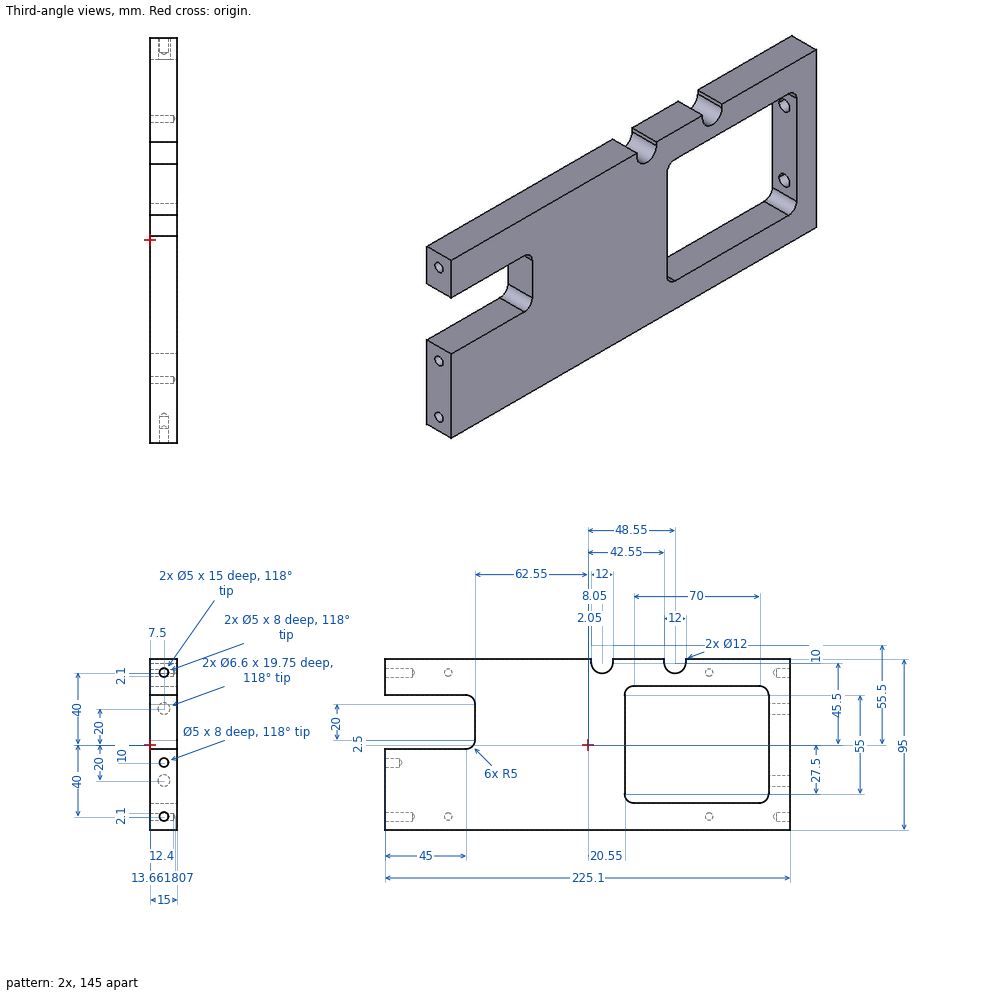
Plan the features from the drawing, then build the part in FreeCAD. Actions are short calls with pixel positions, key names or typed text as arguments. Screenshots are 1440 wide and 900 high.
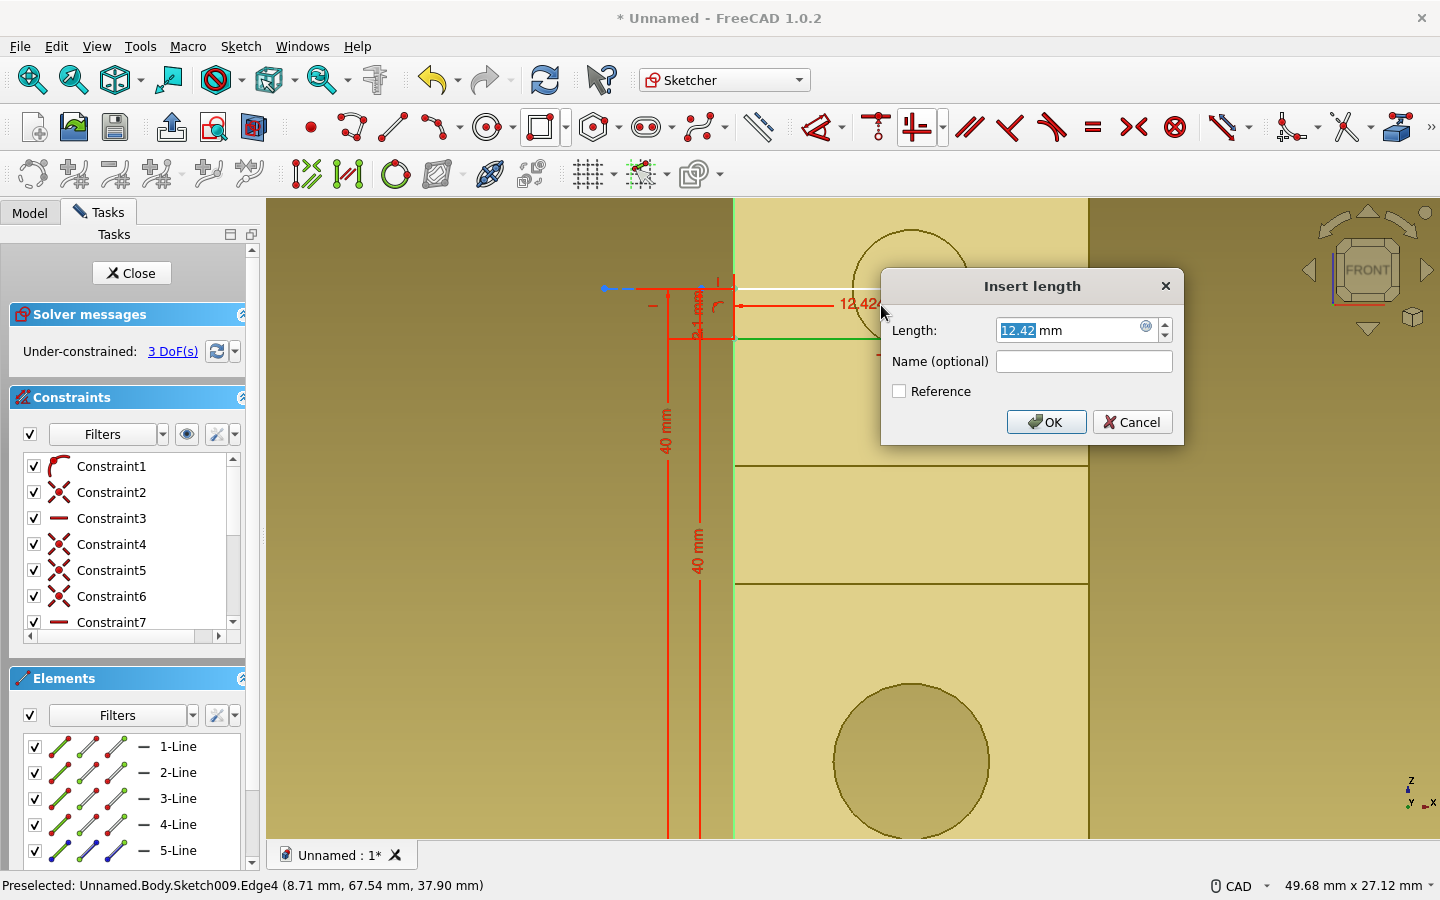
text(12.4)
key(Return)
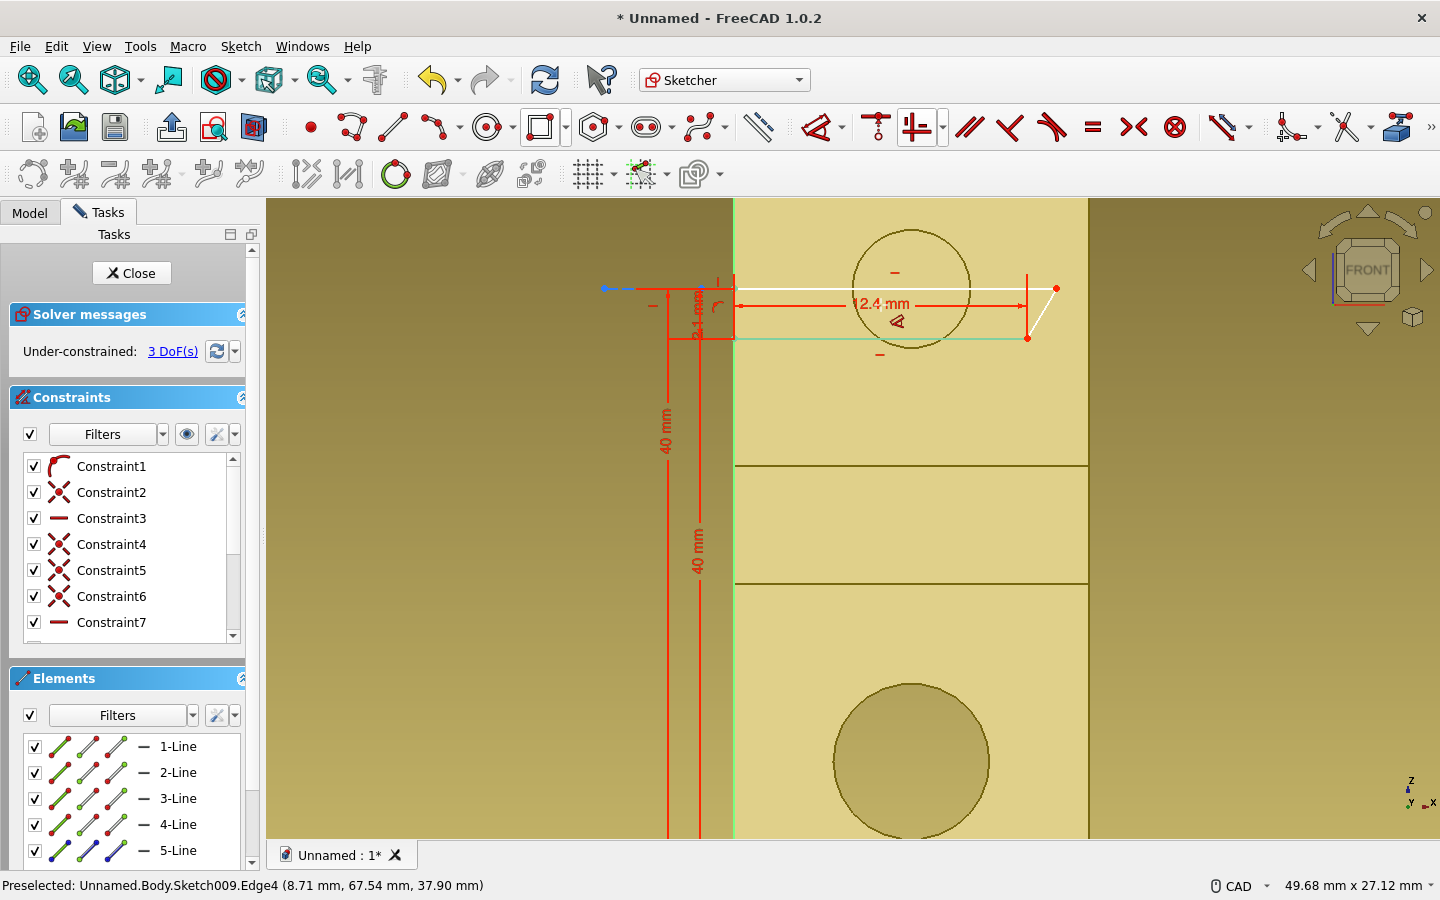
click(831, 289)
click(895, 255)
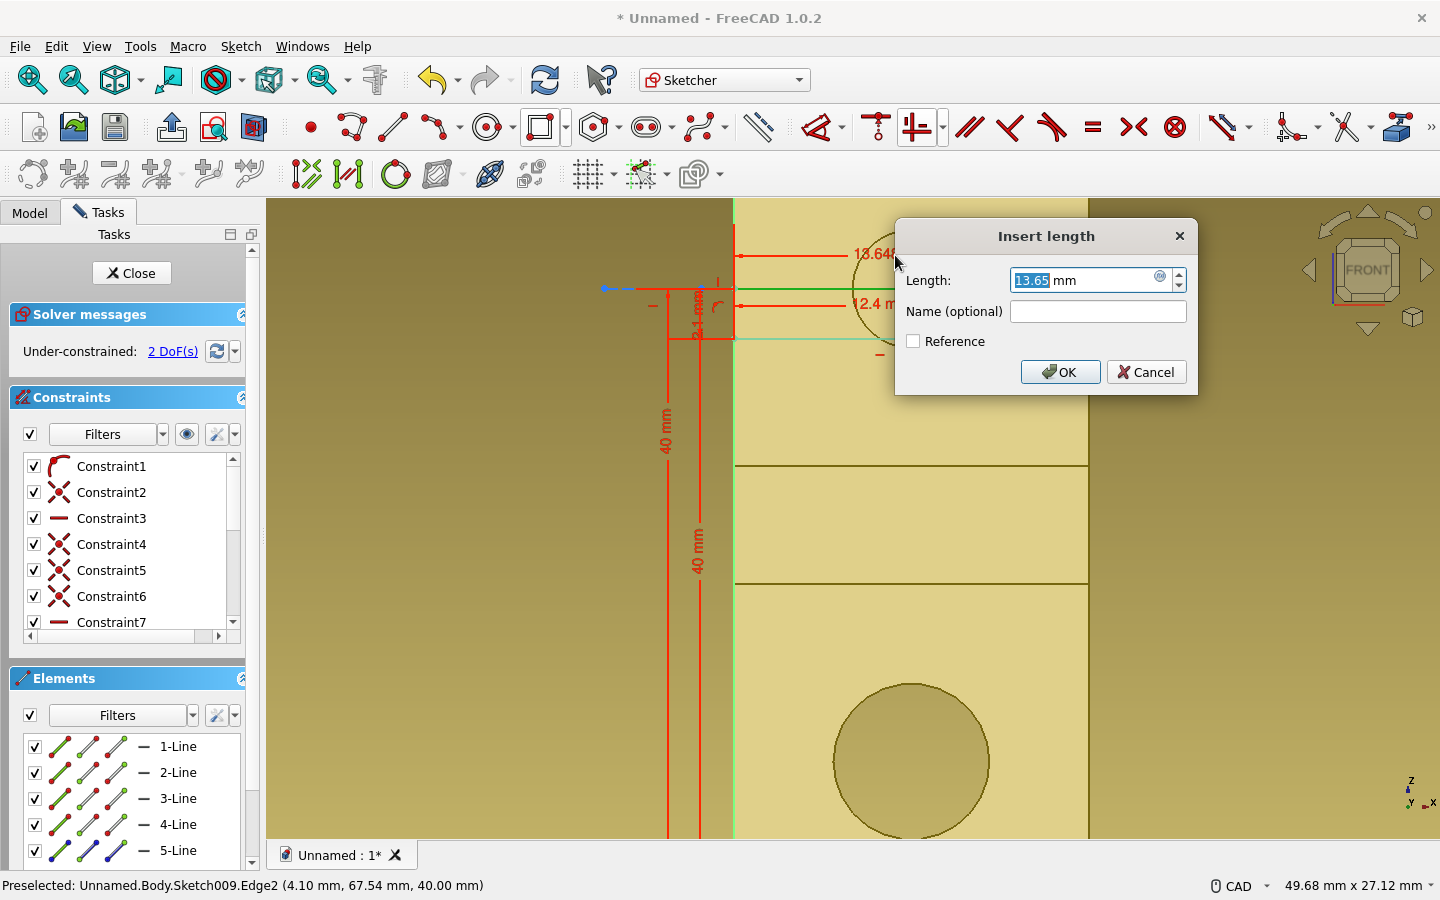
text(13.661807)
key(Return)
key(Escape)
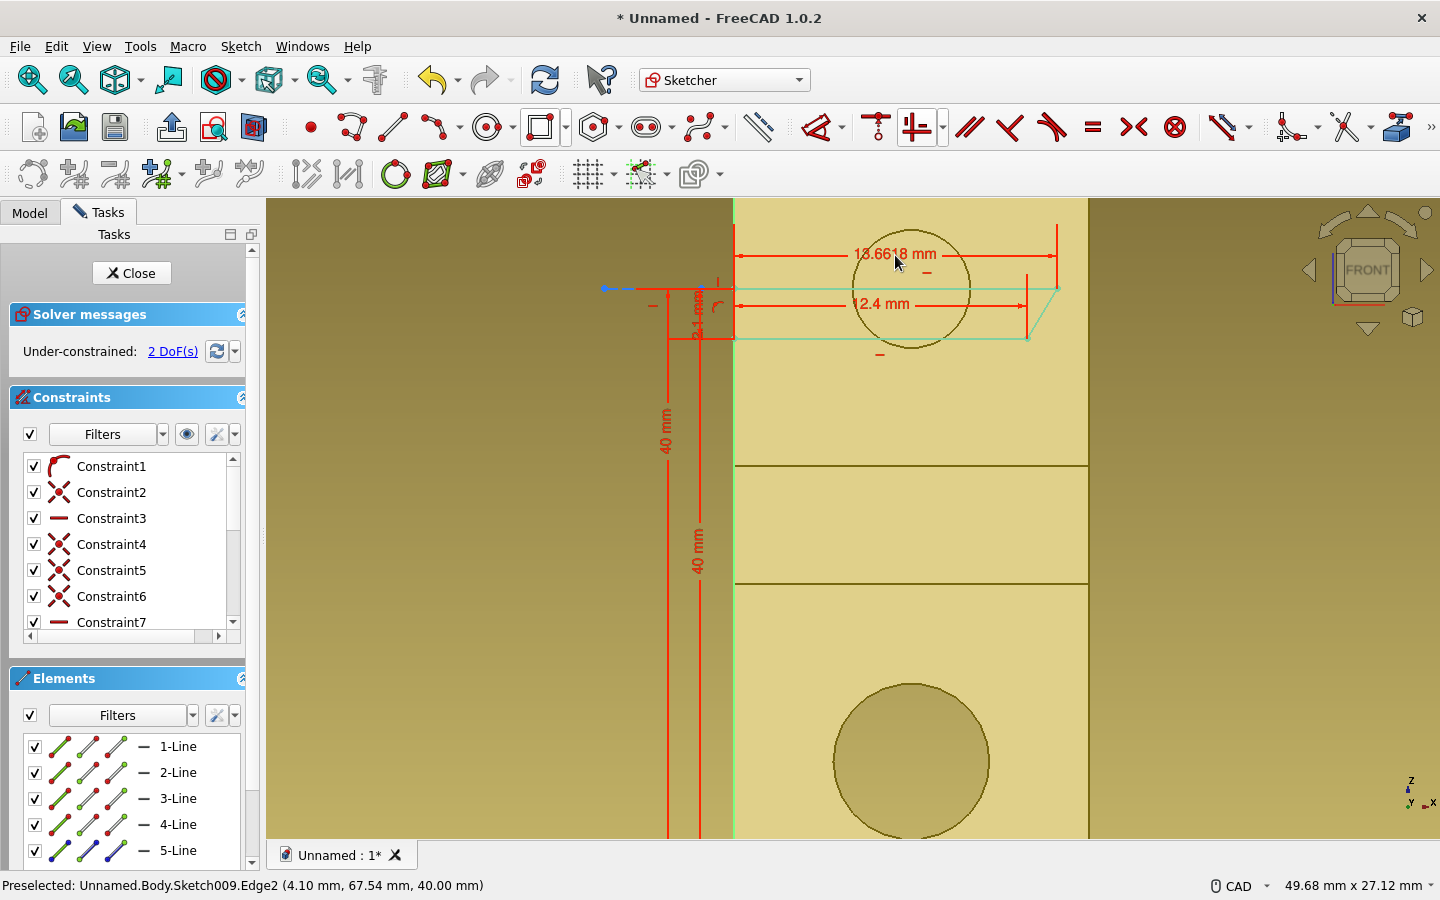
click(132, 273)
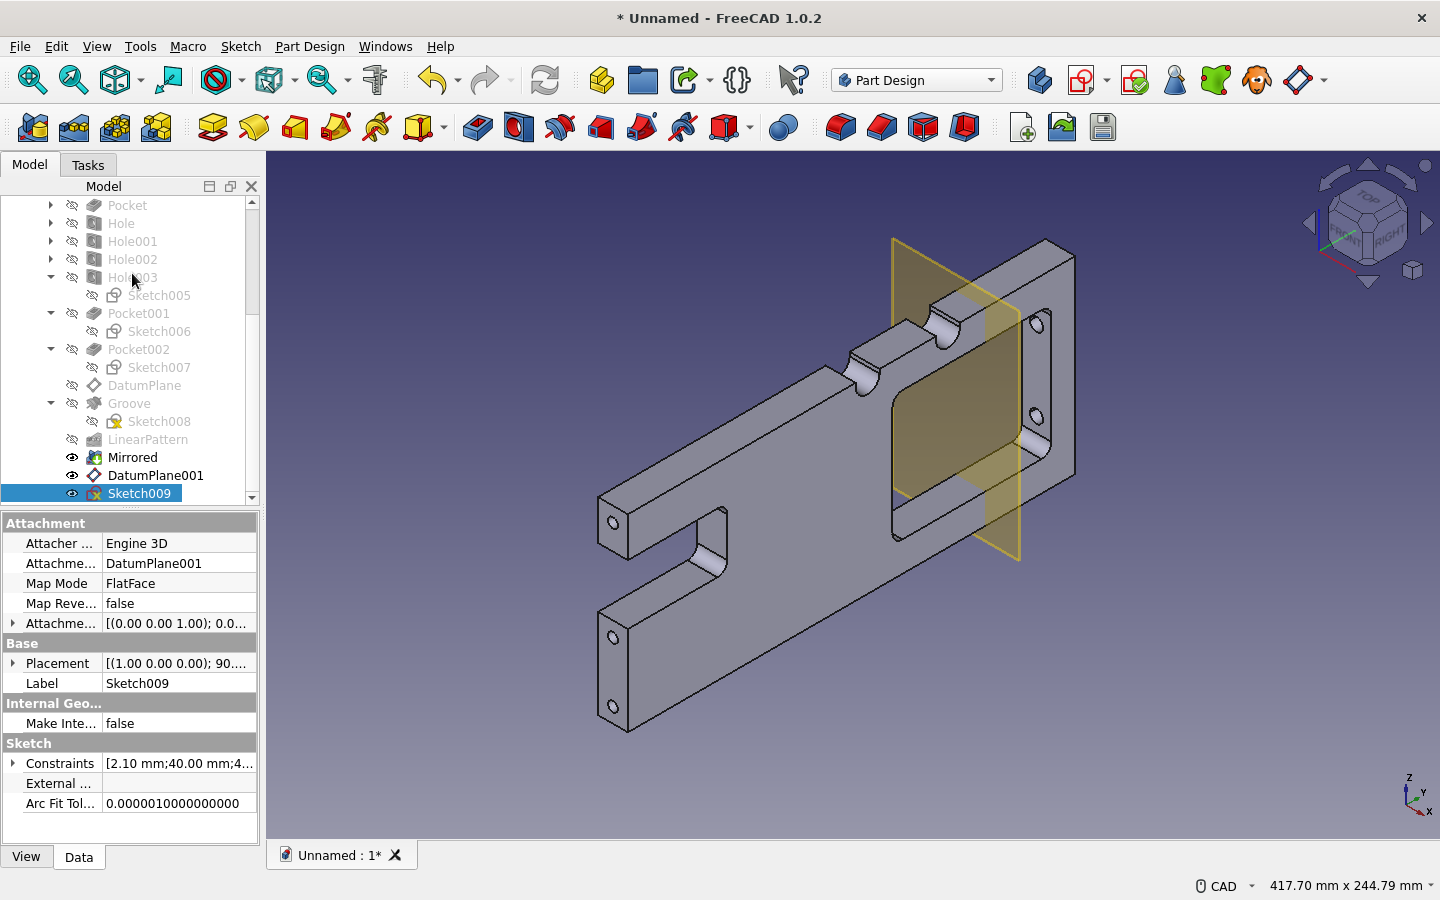
click(560, 128)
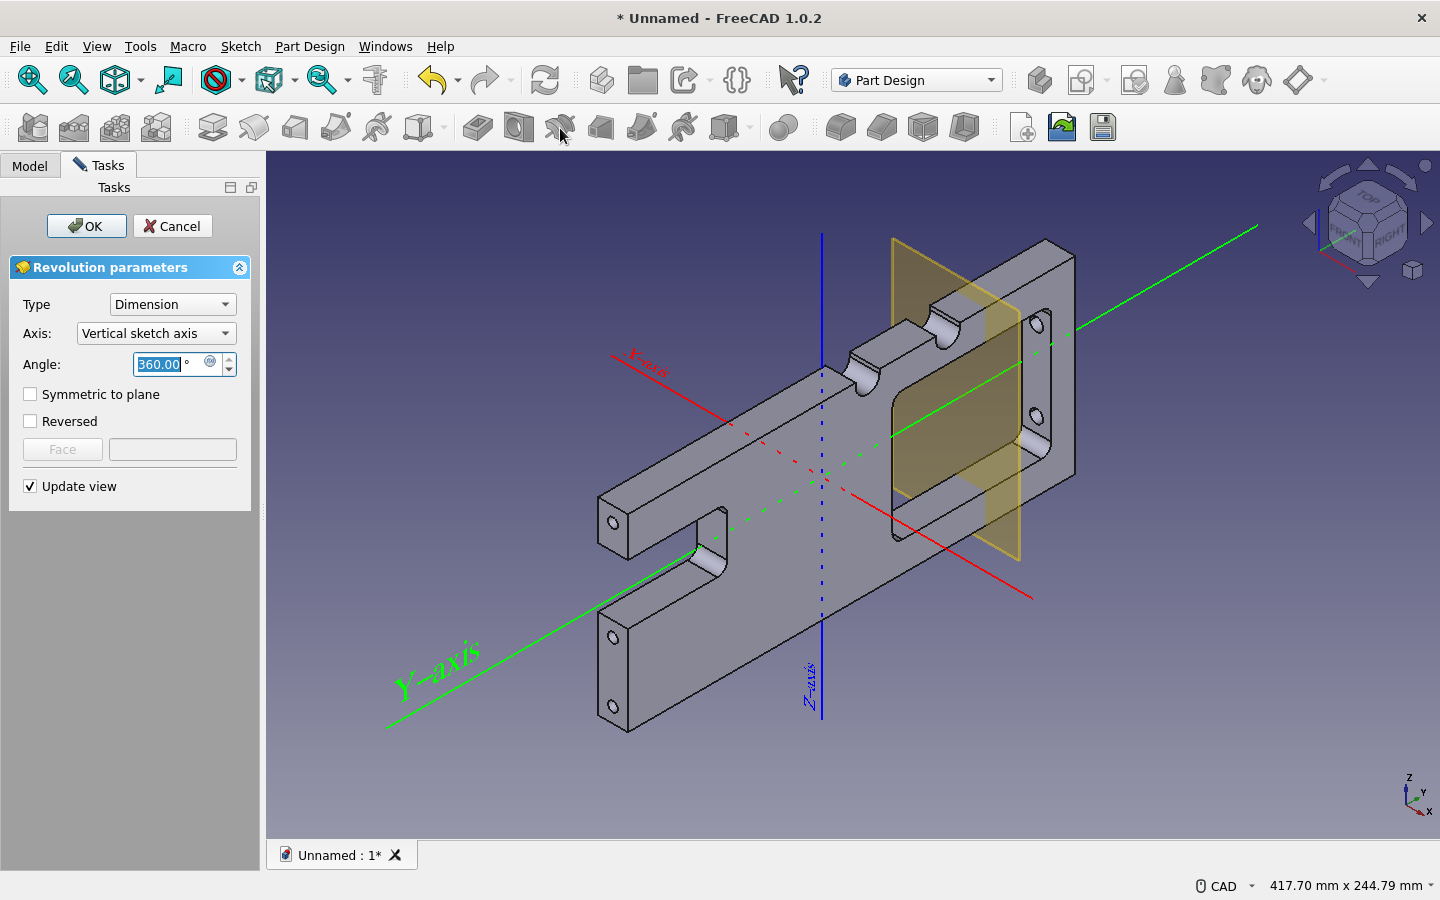
click(157, 334)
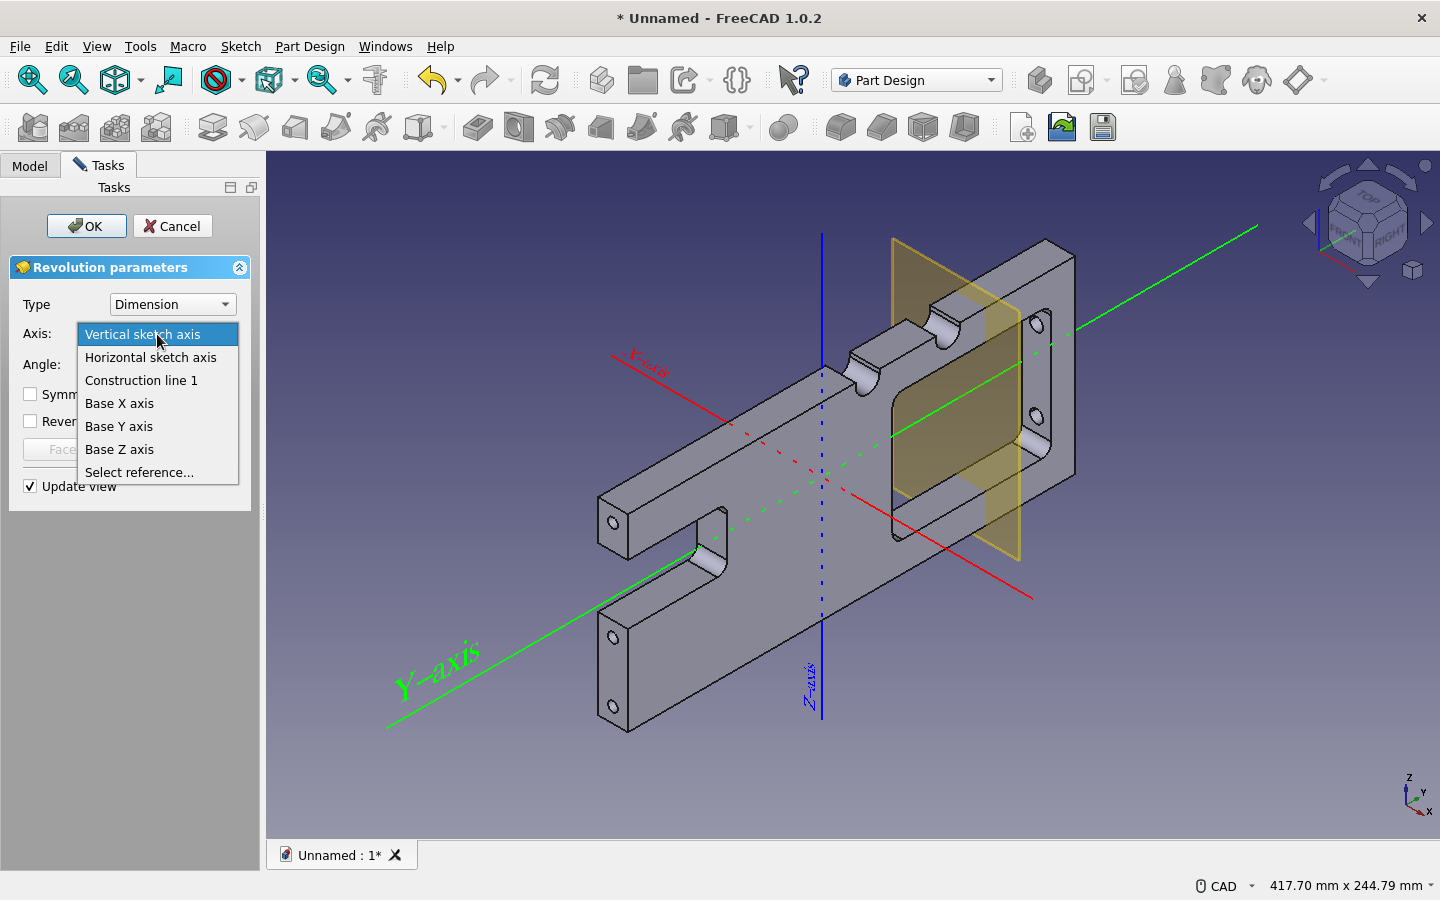
click(156, 380)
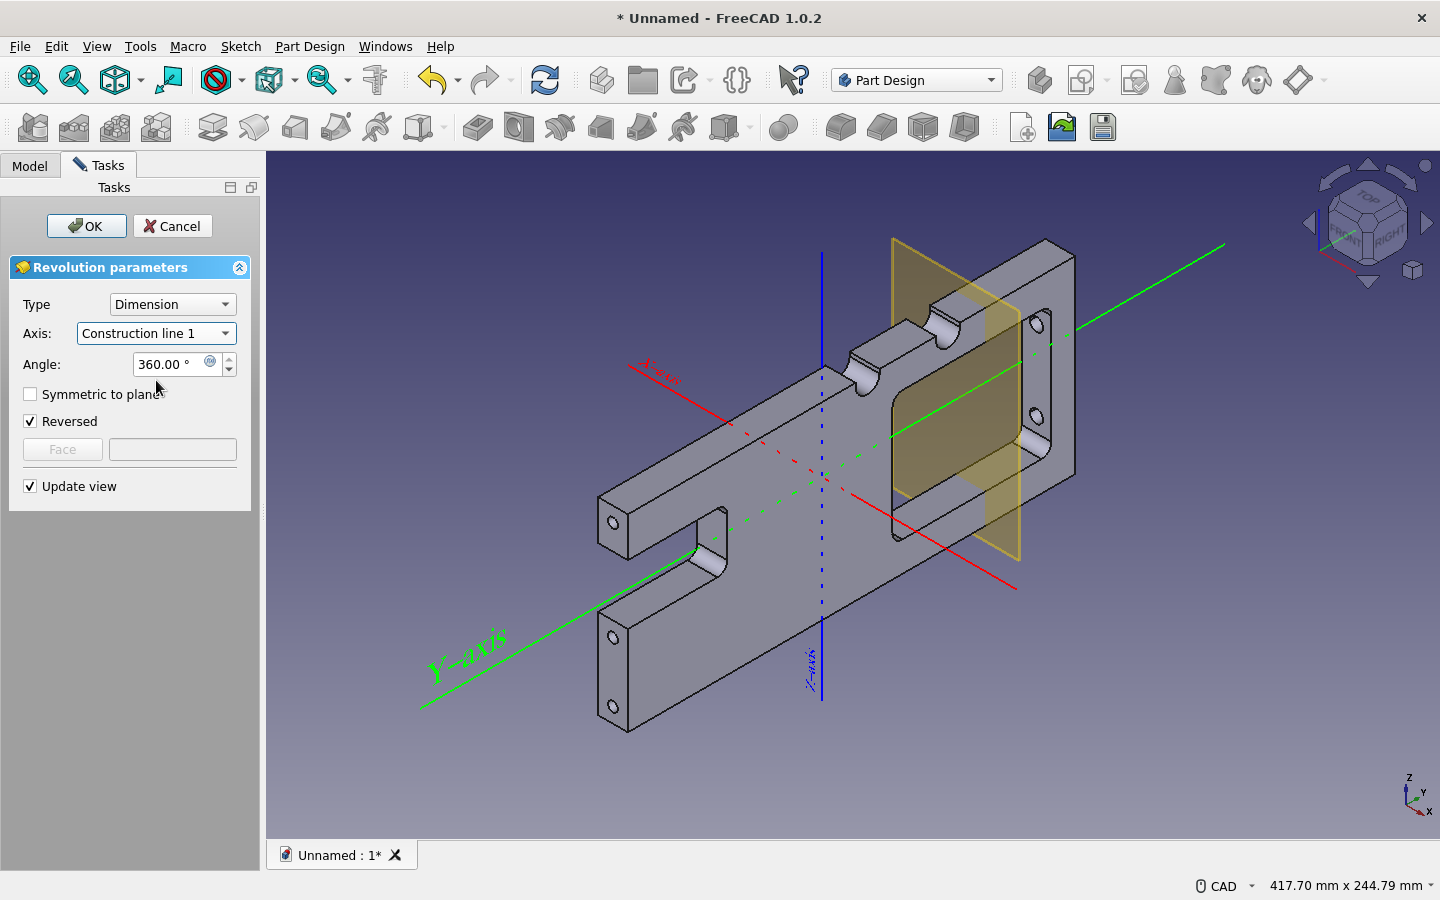
click(87, 226)